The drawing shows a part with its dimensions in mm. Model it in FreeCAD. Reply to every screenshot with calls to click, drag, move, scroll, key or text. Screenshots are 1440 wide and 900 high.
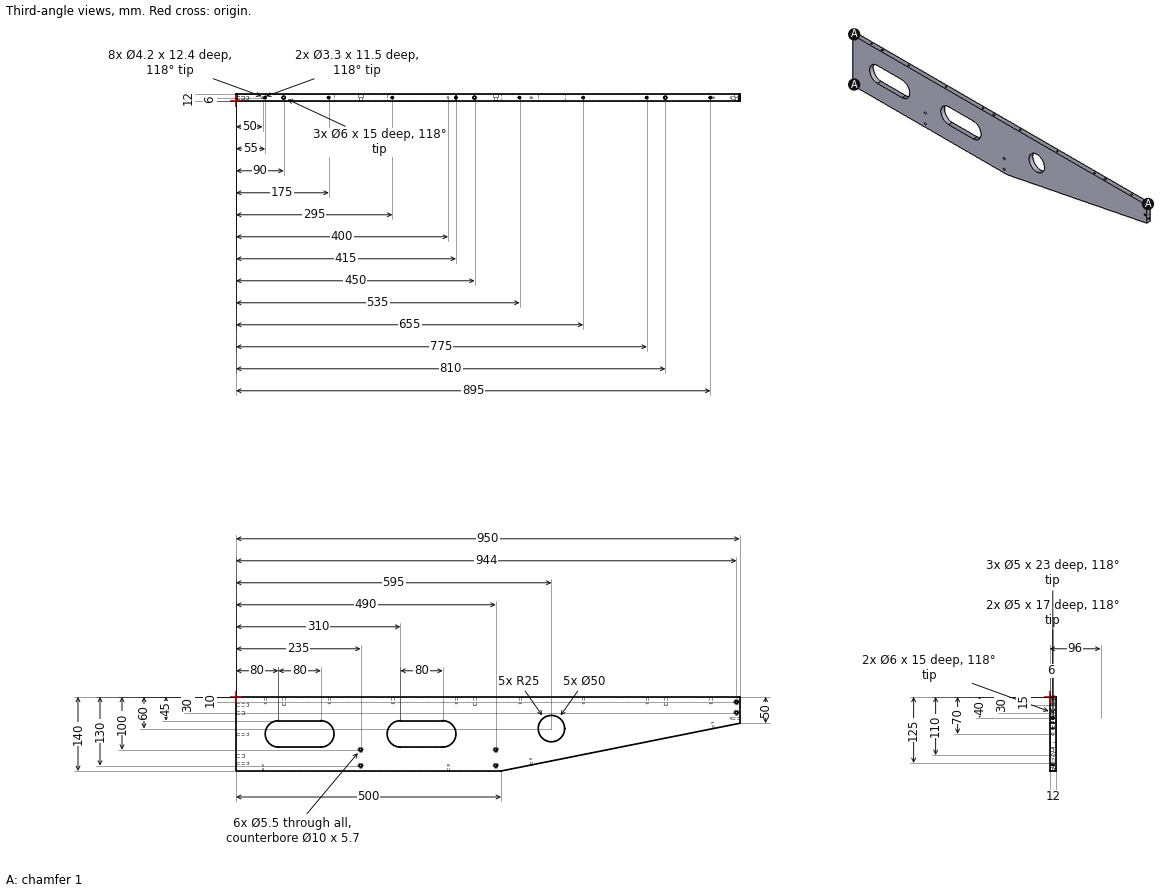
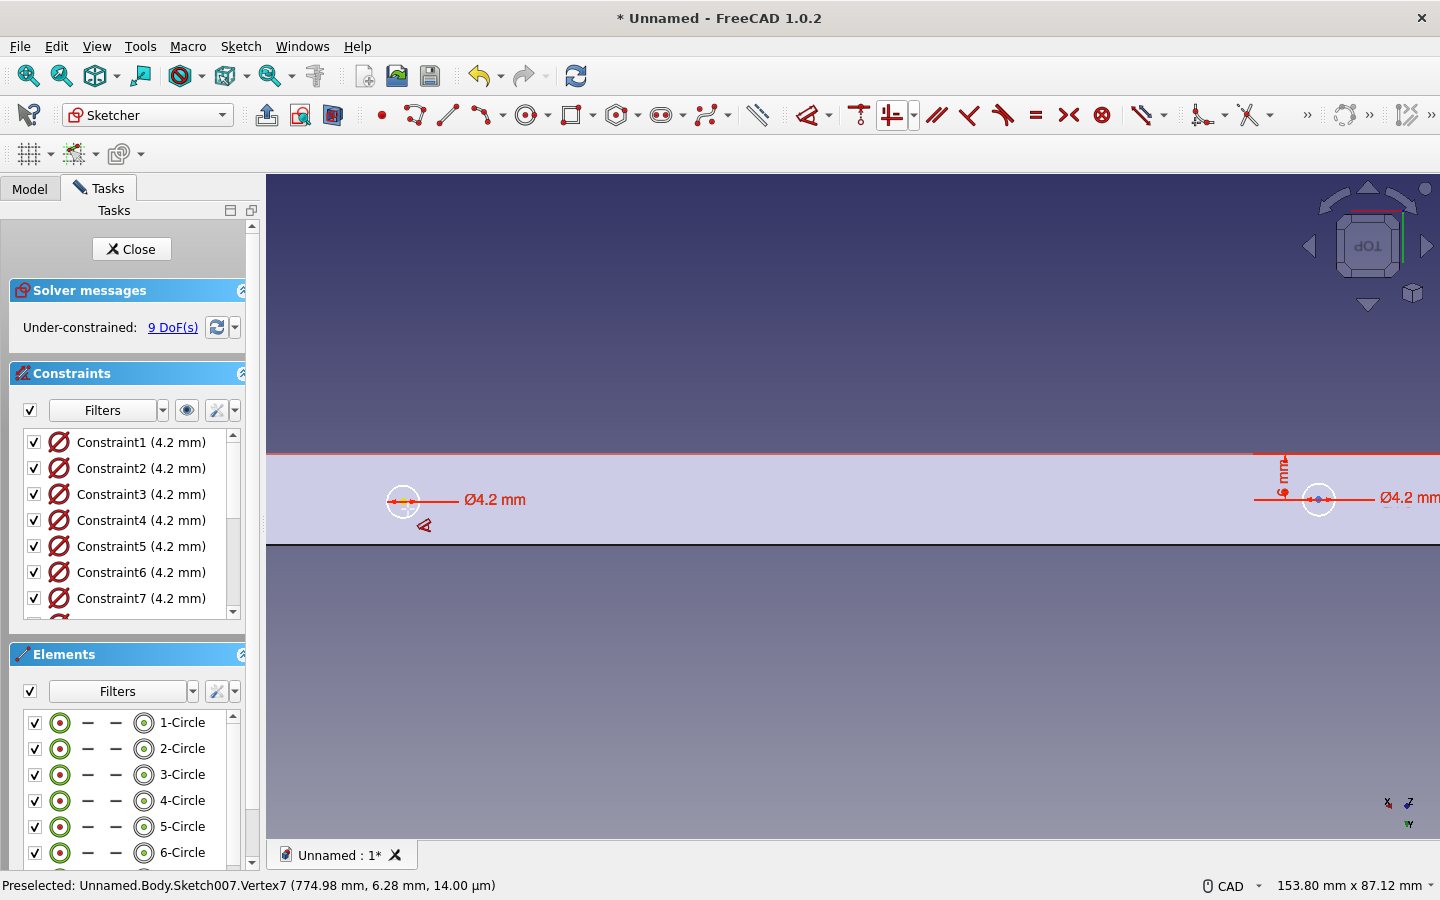
click(403, 502)
click(369, 478)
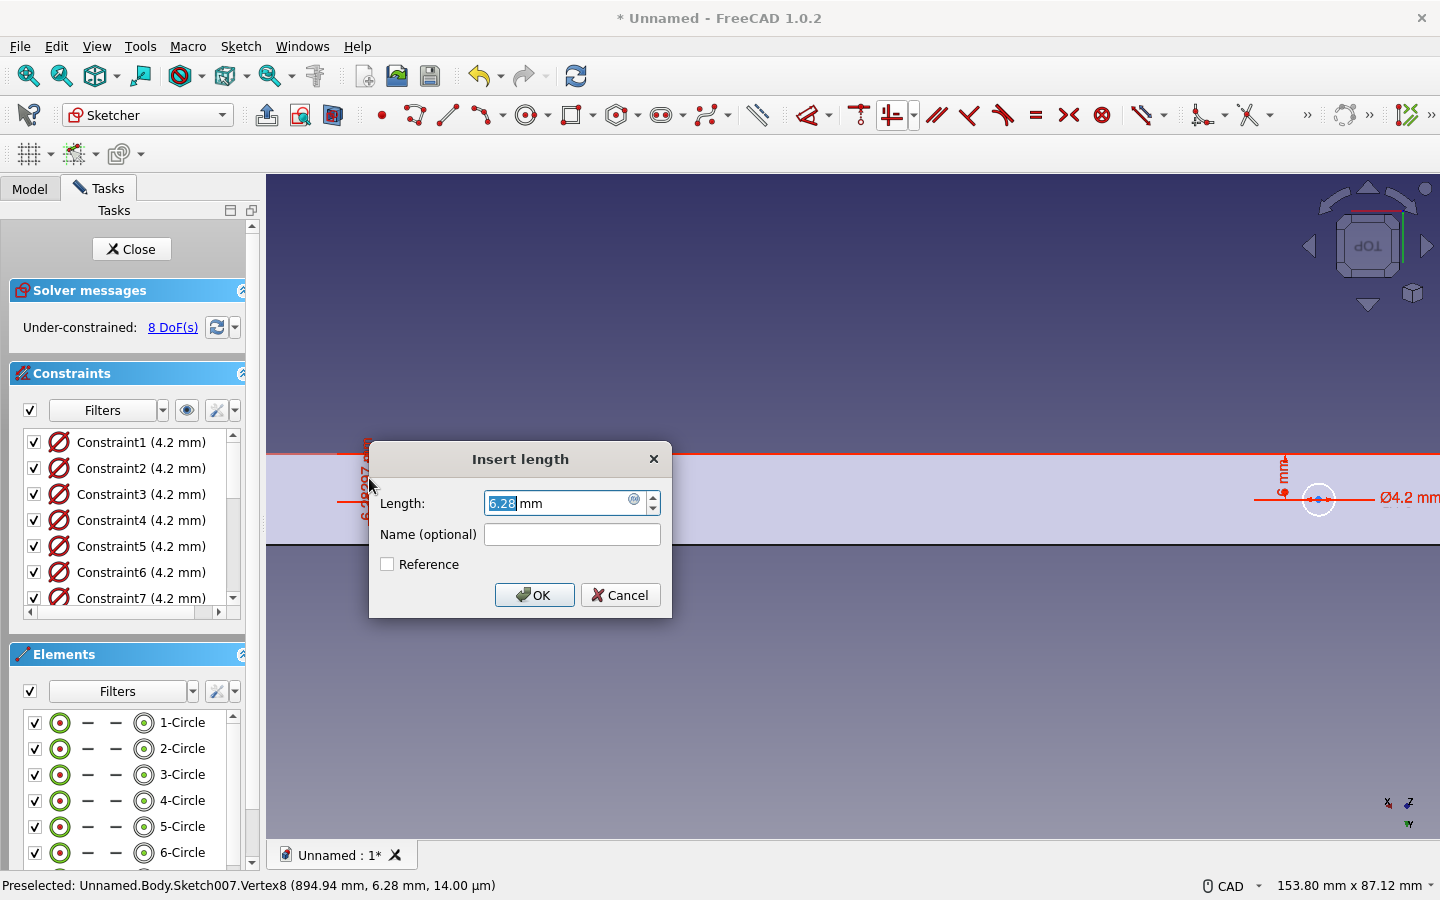
text(6)
key(Return)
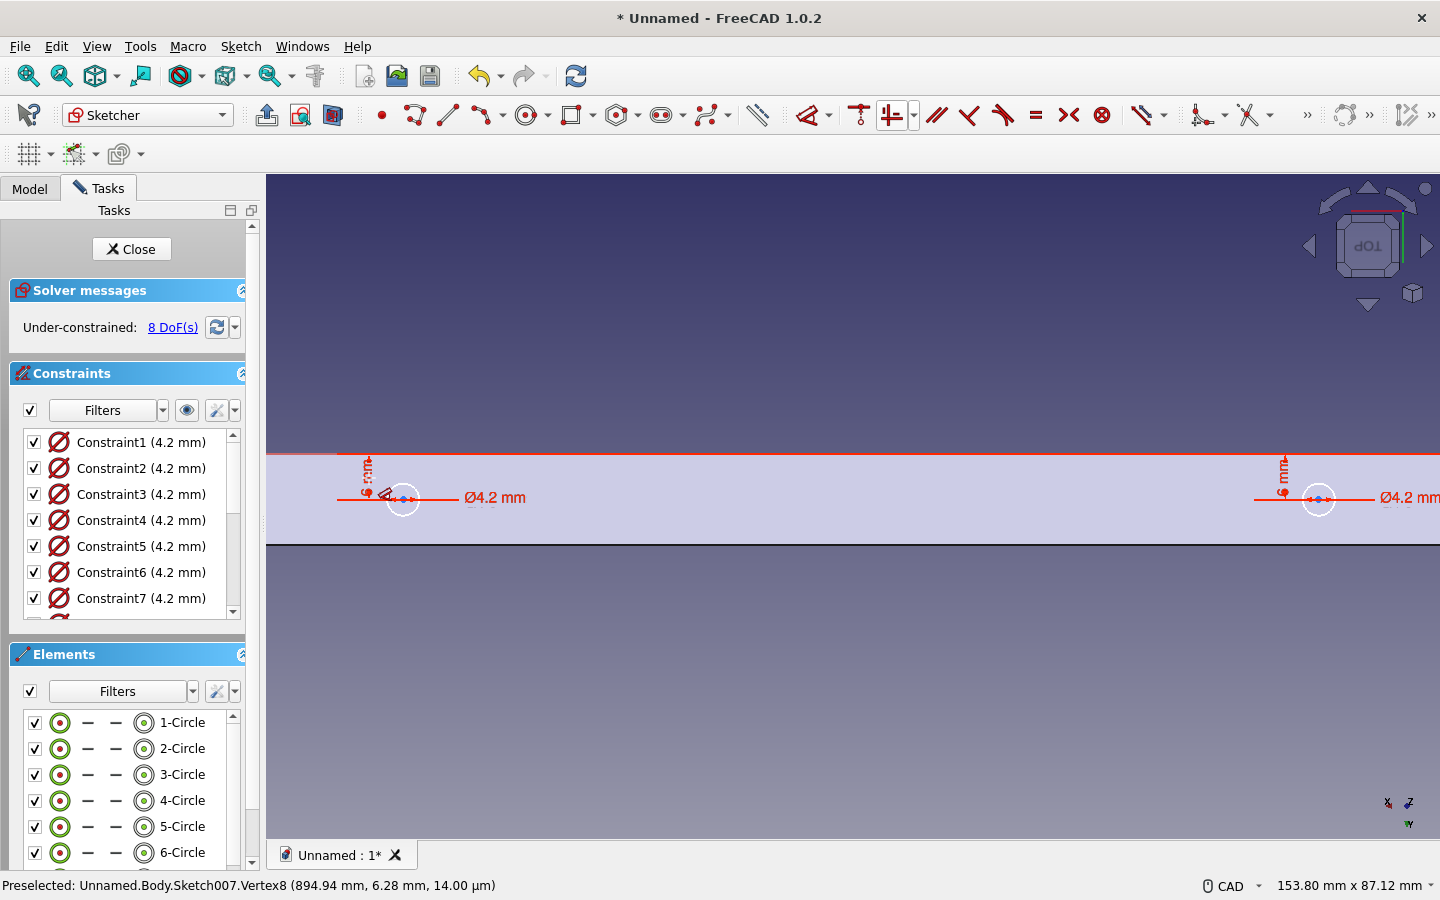
scroll(407, 509, down, 11)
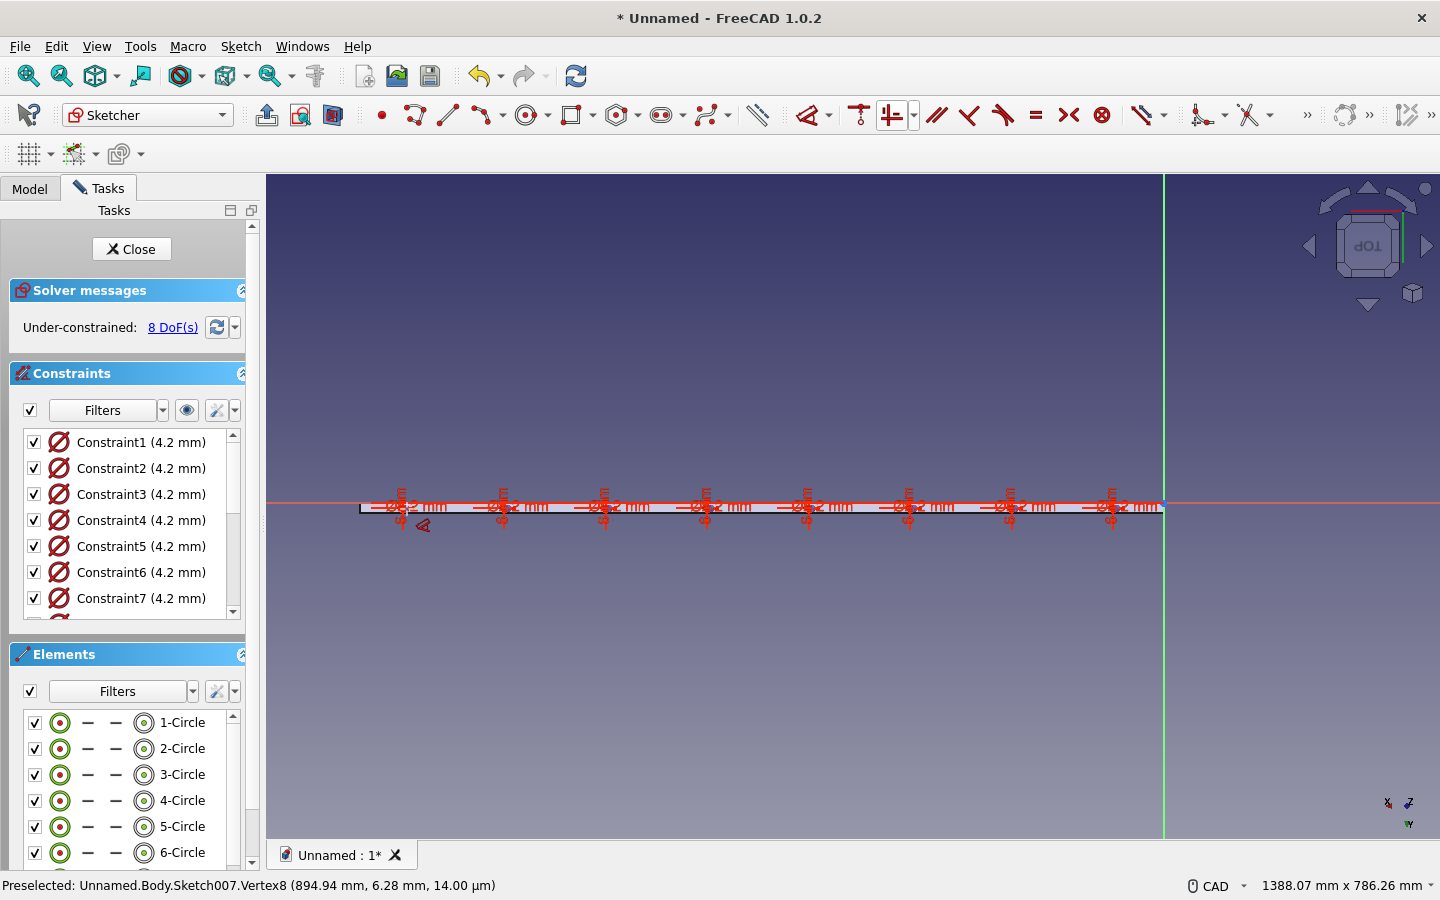
click(1117, 508)
click(1140, 469)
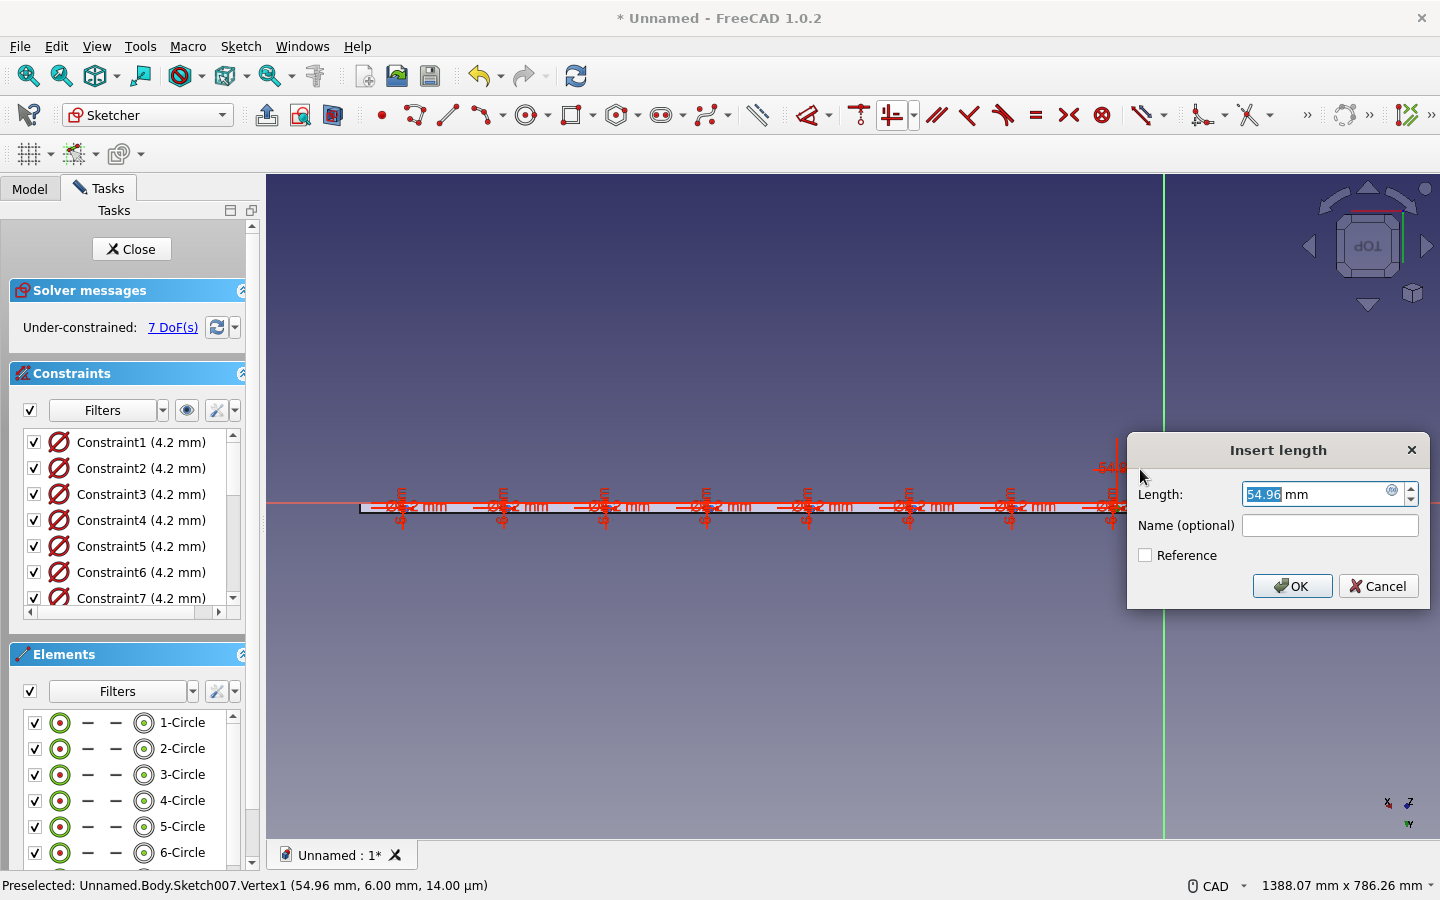
text(55)
key(Return)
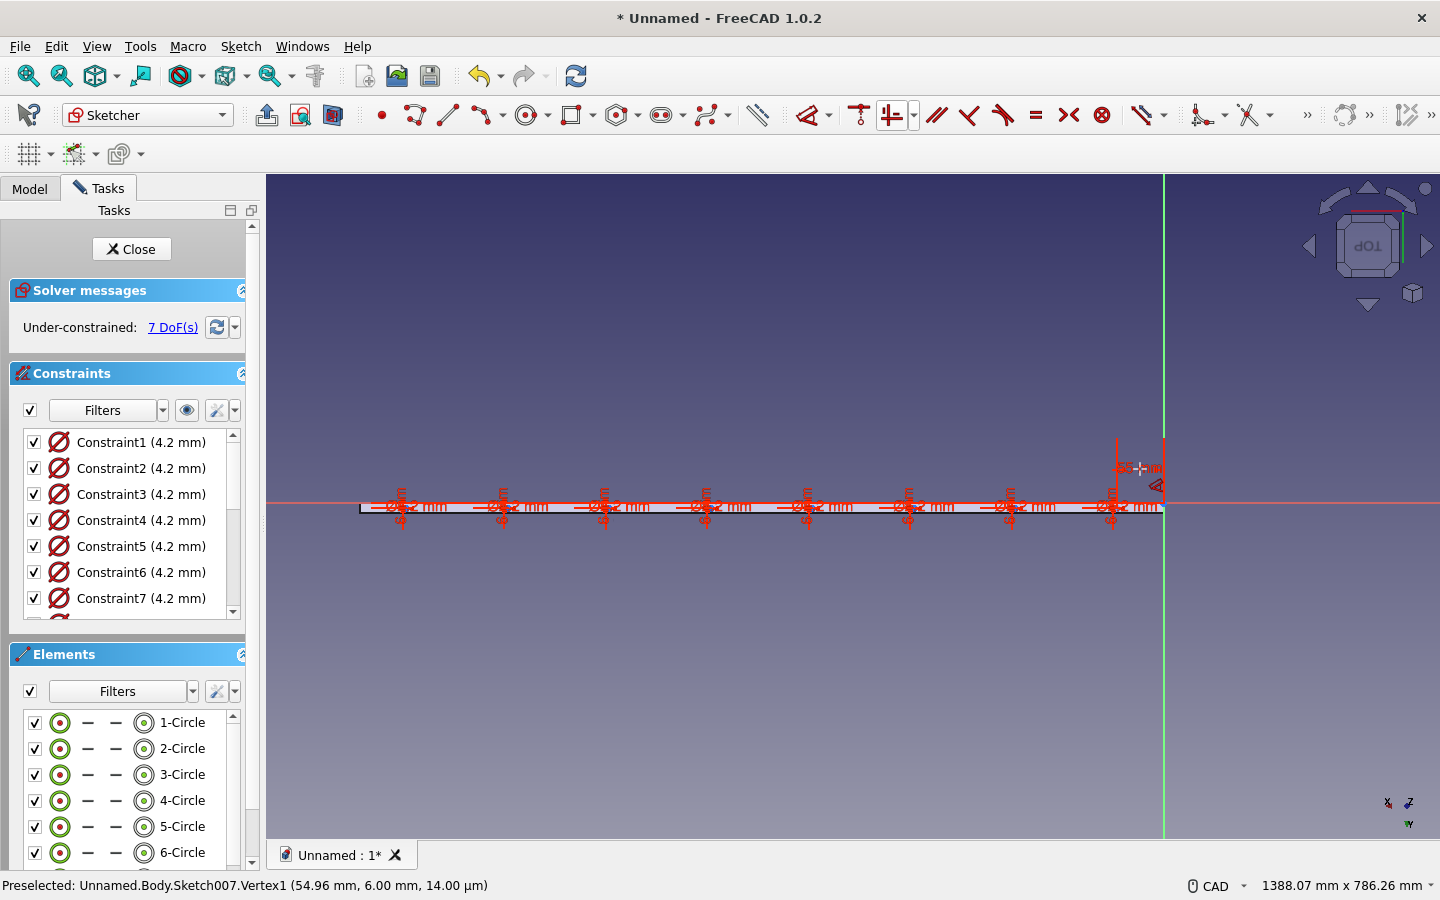
click(1016, 508)
click(1056, 469)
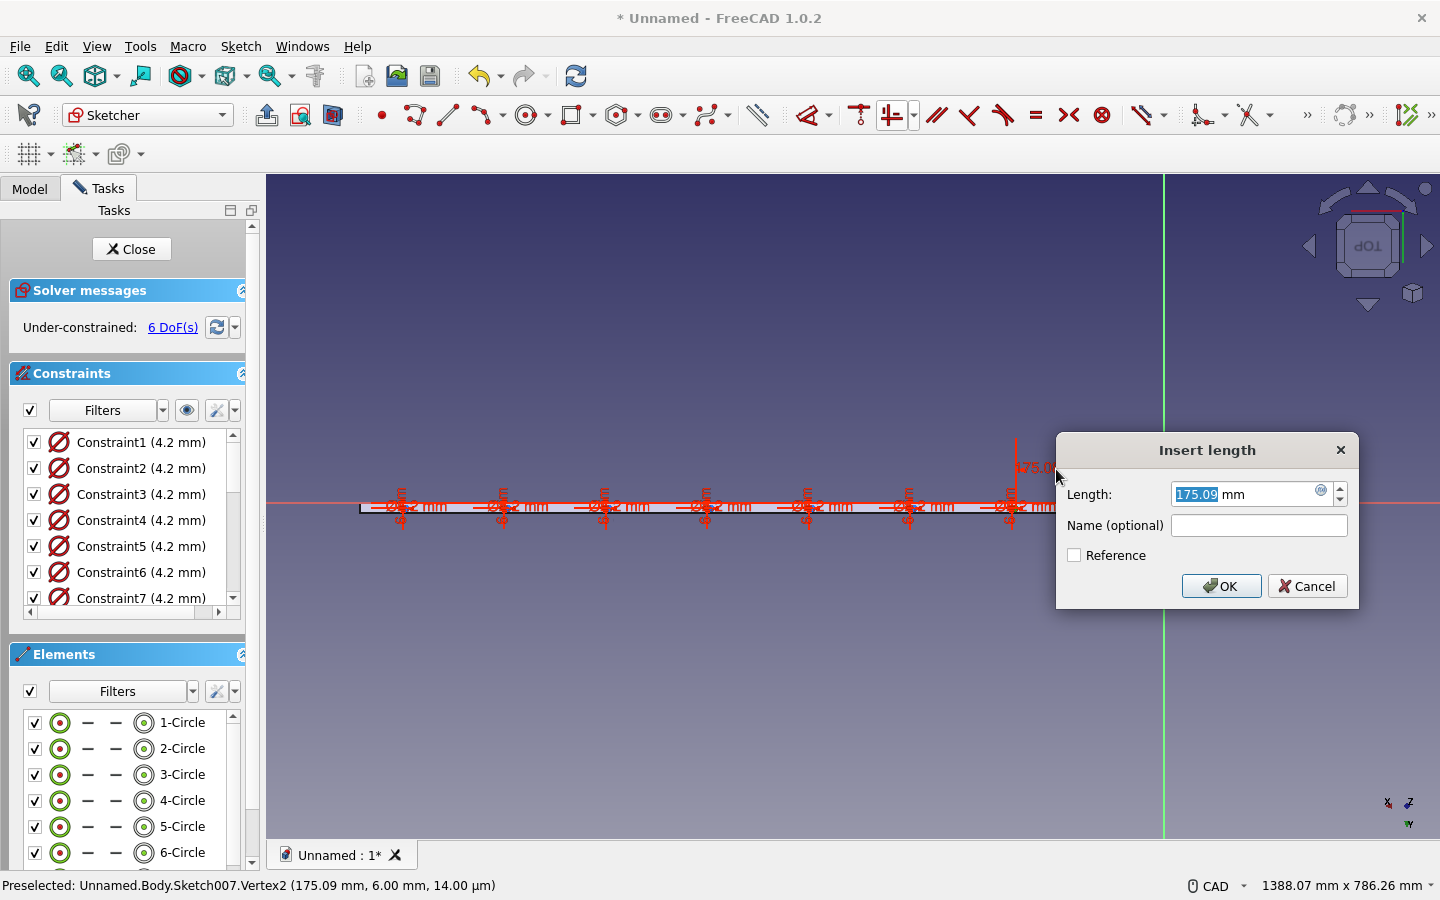
text(175)
key(Return)